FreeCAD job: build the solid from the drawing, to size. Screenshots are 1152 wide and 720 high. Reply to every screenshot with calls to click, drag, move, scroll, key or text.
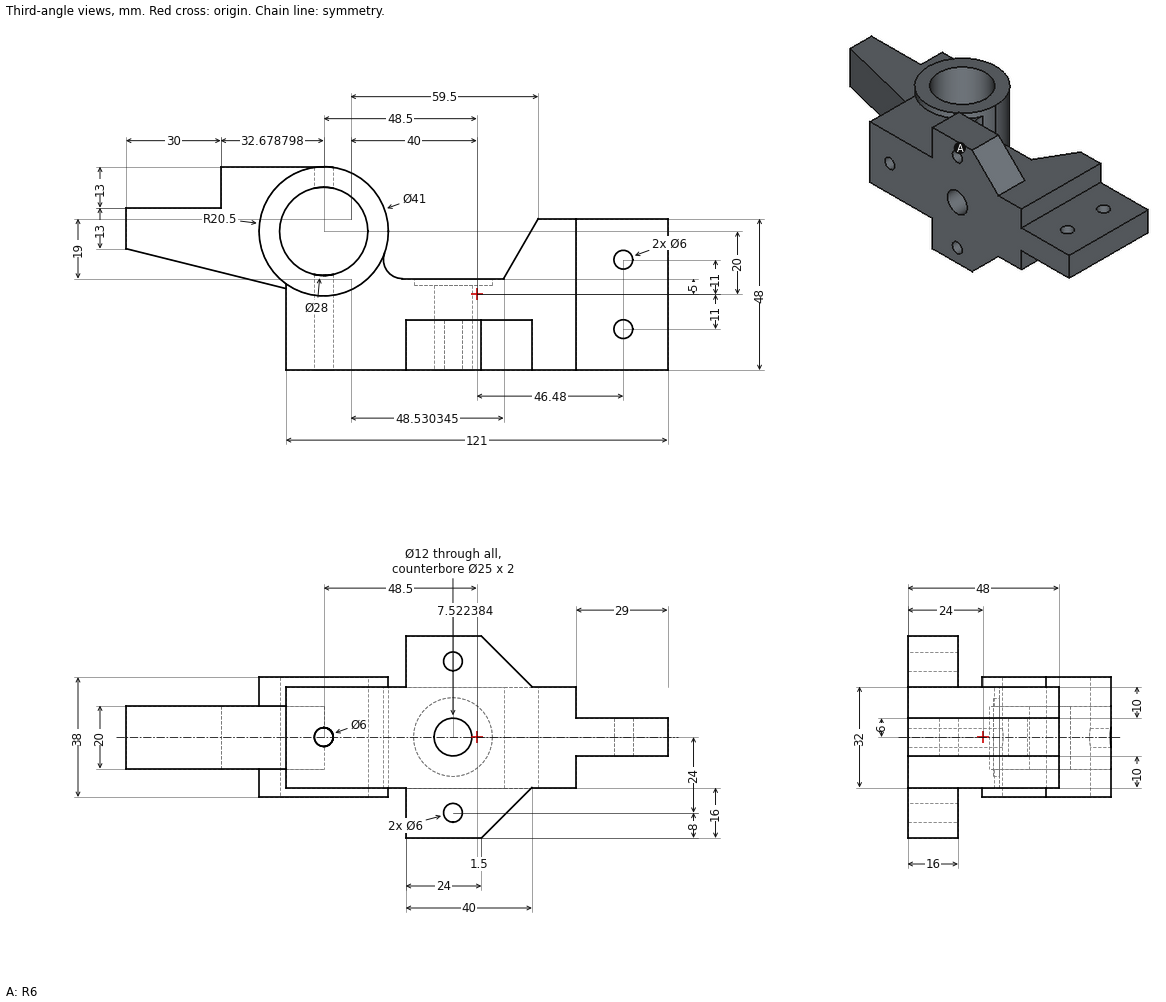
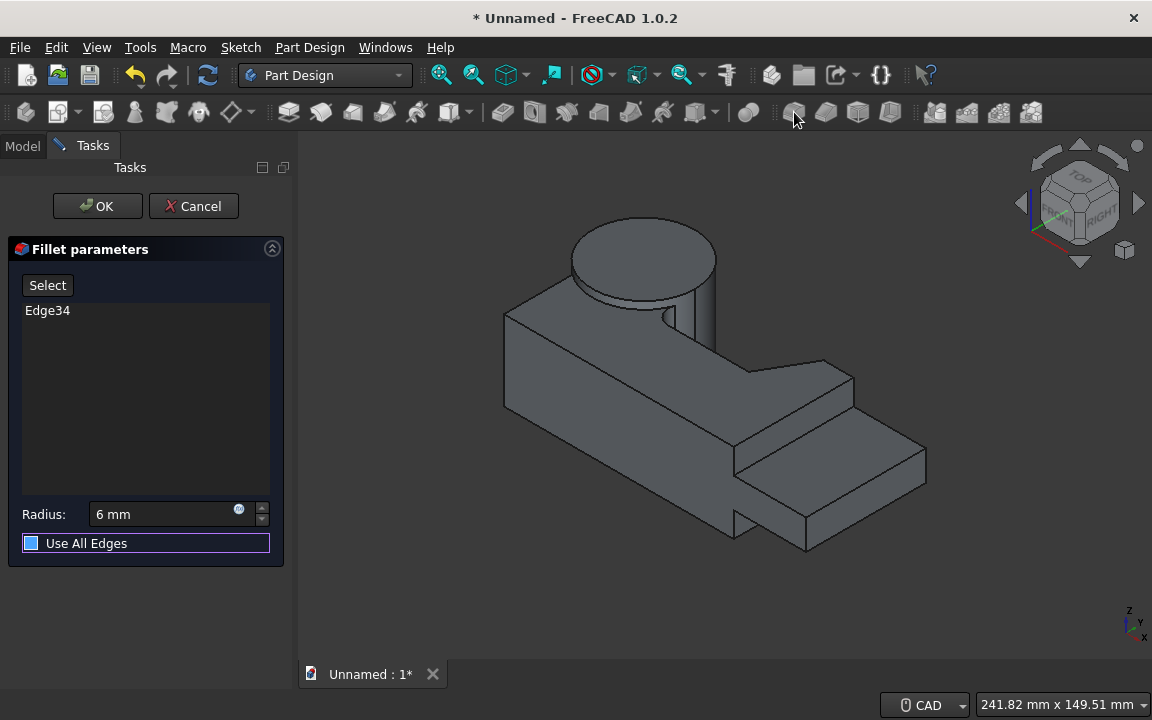
click(98, 206)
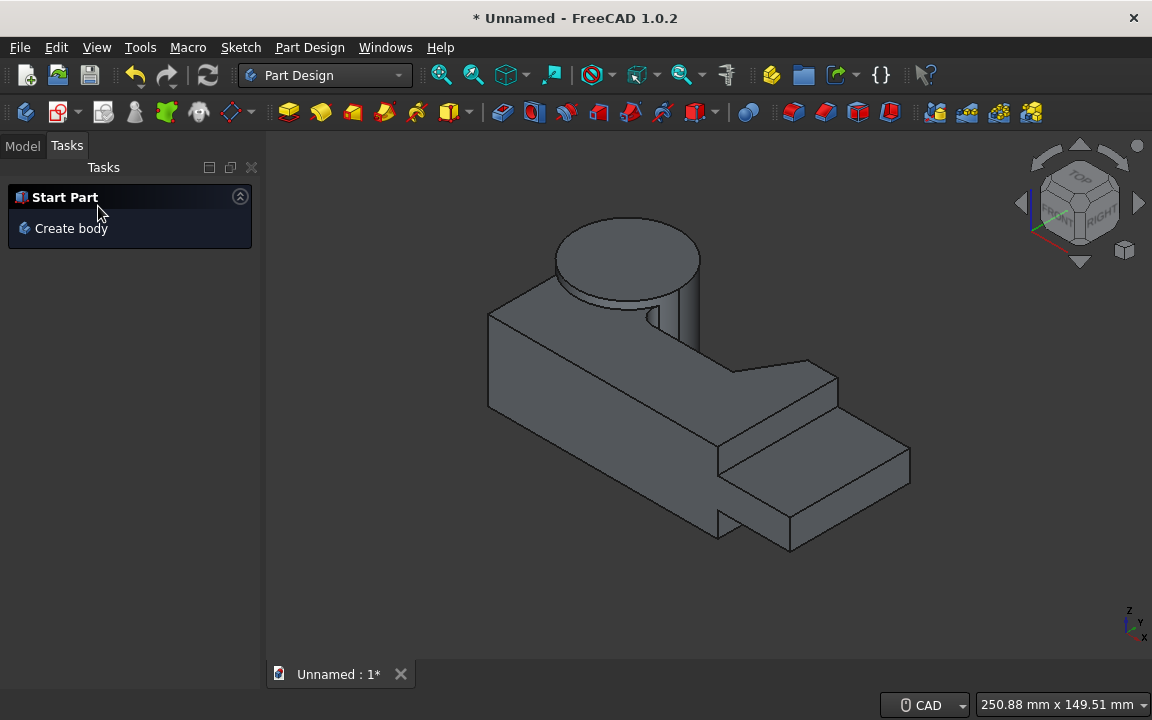
click(58, 112)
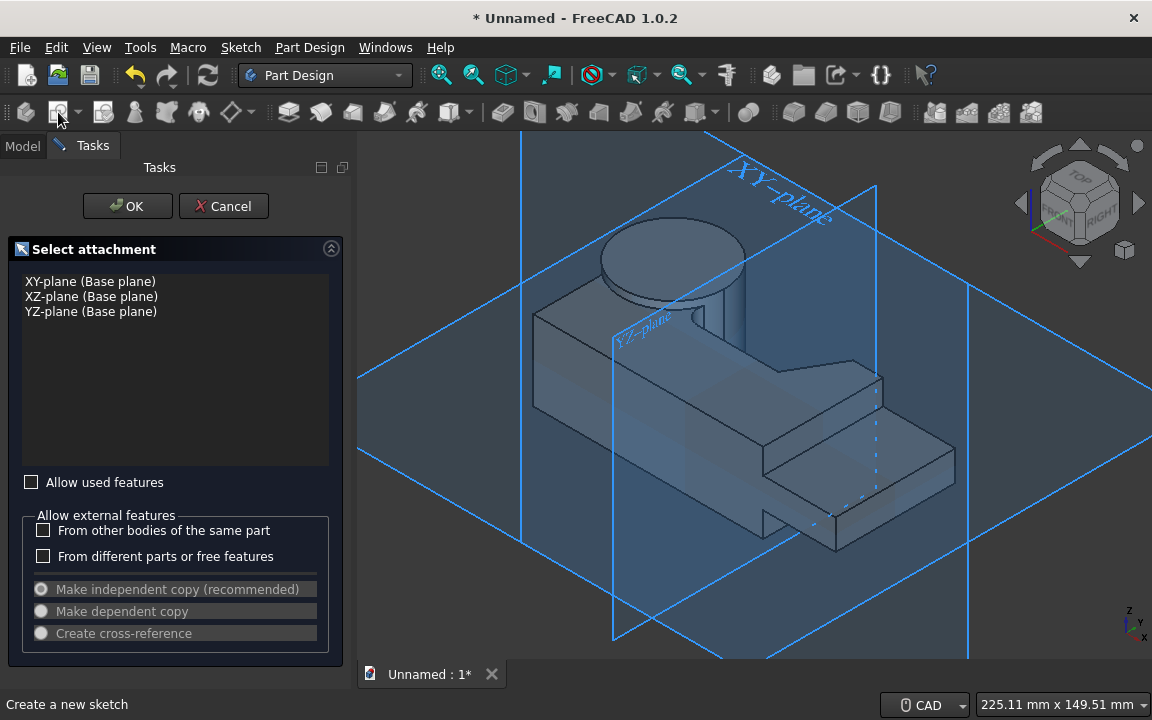
click(82, 282)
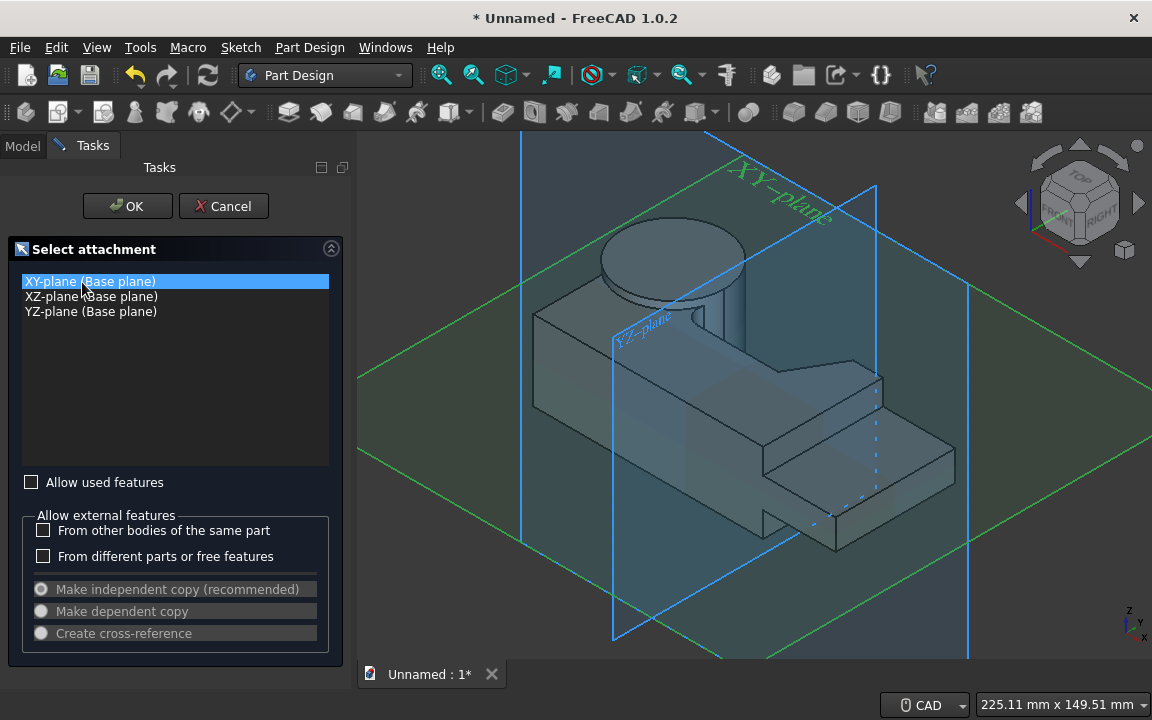
click(128, 206)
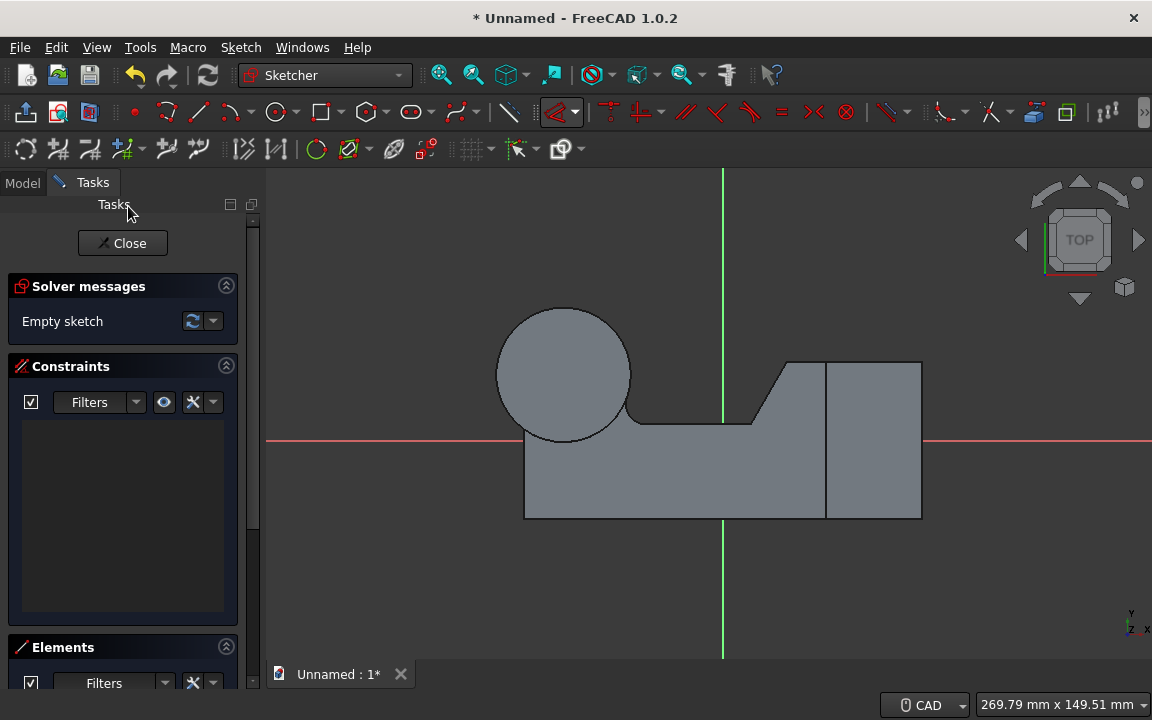
key(q)
key(s)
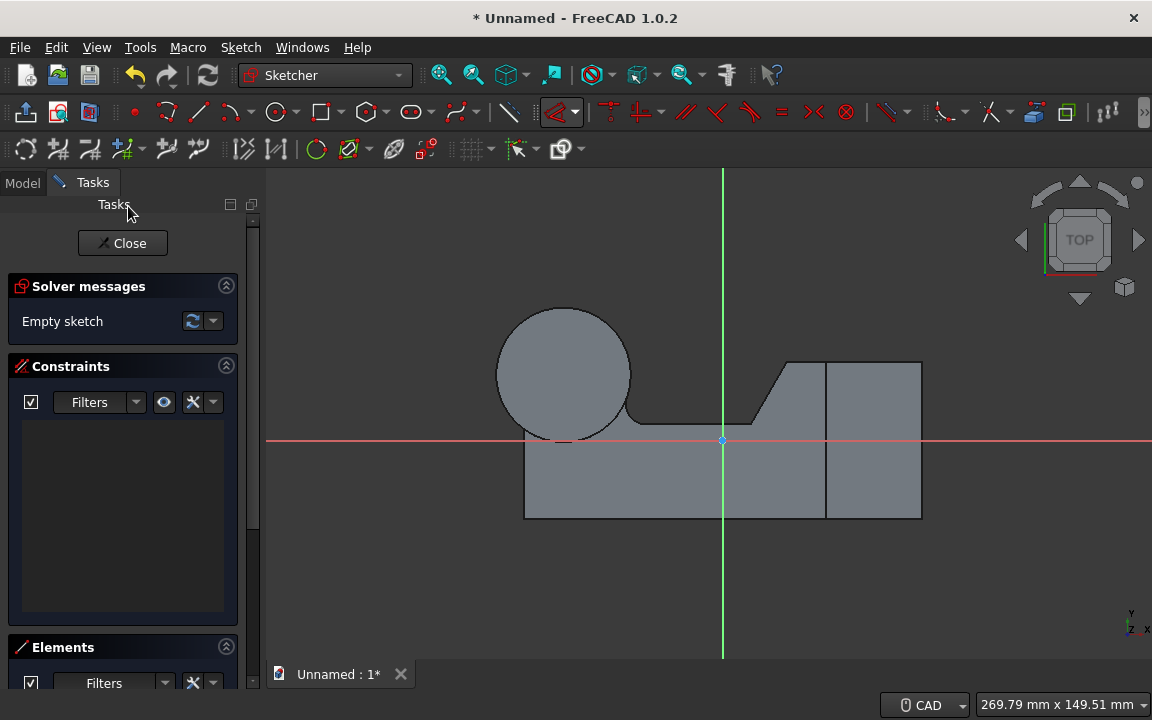
key(g)
key(m)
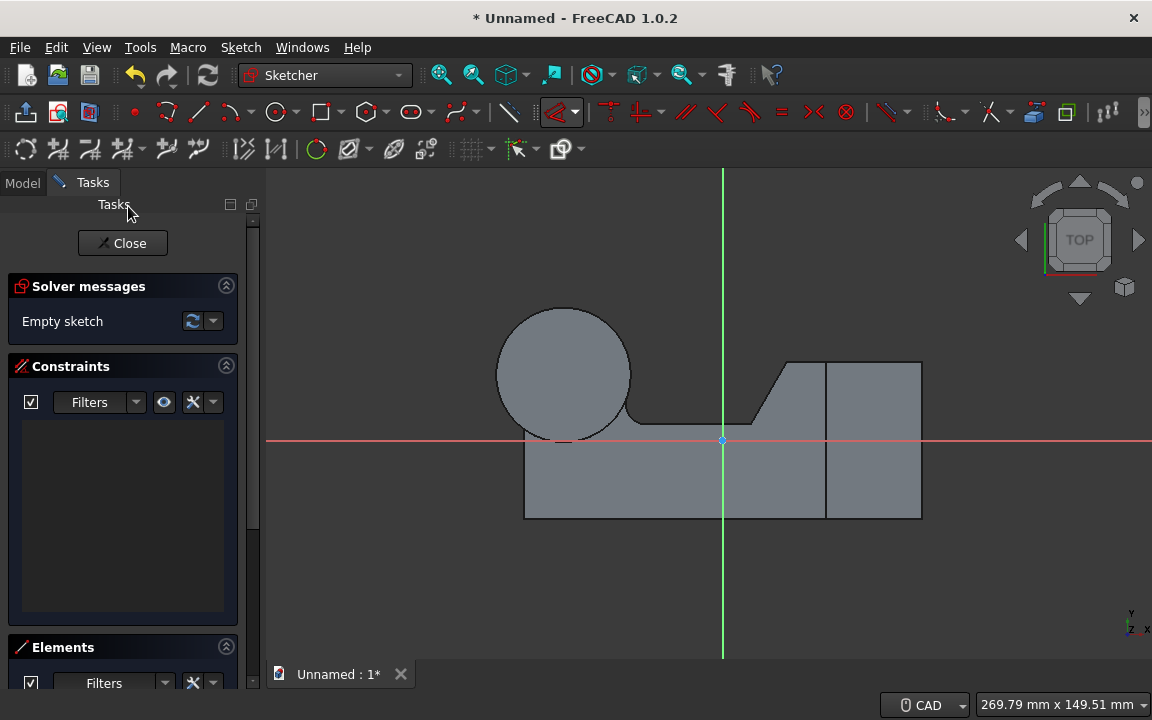
click(564, 308)
click(456, 308)
click(456, 350)
click(358, 350)
click(358, 393)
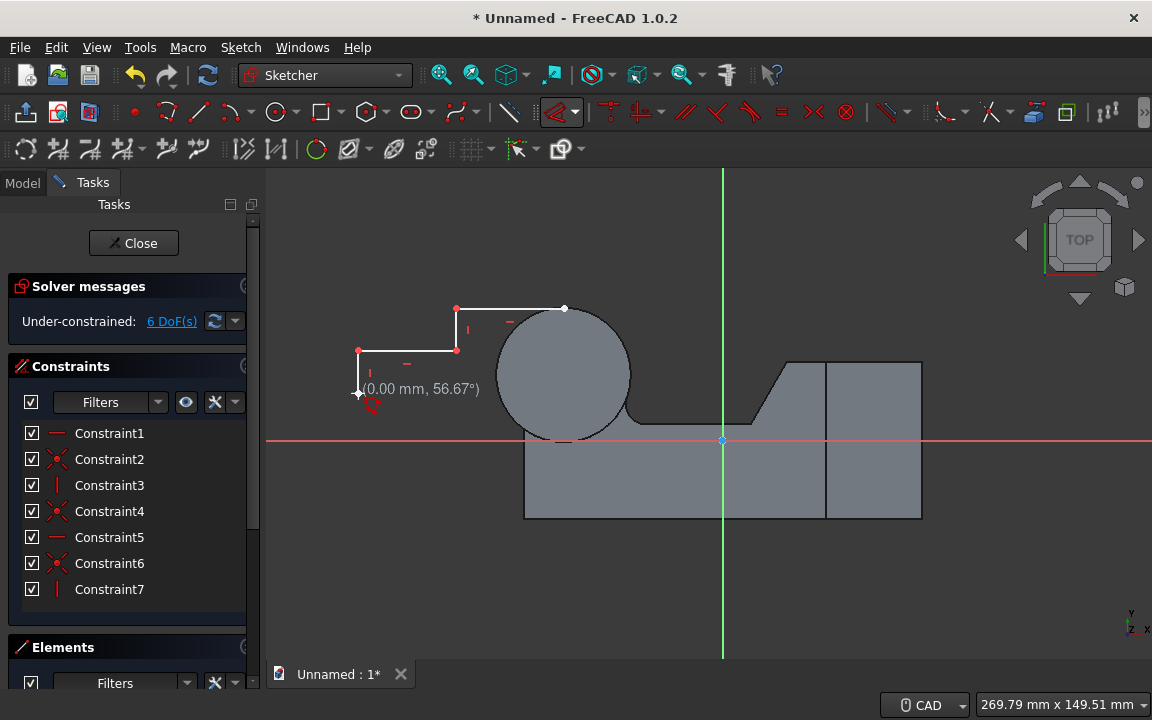
scroll(547, 440, up, 19)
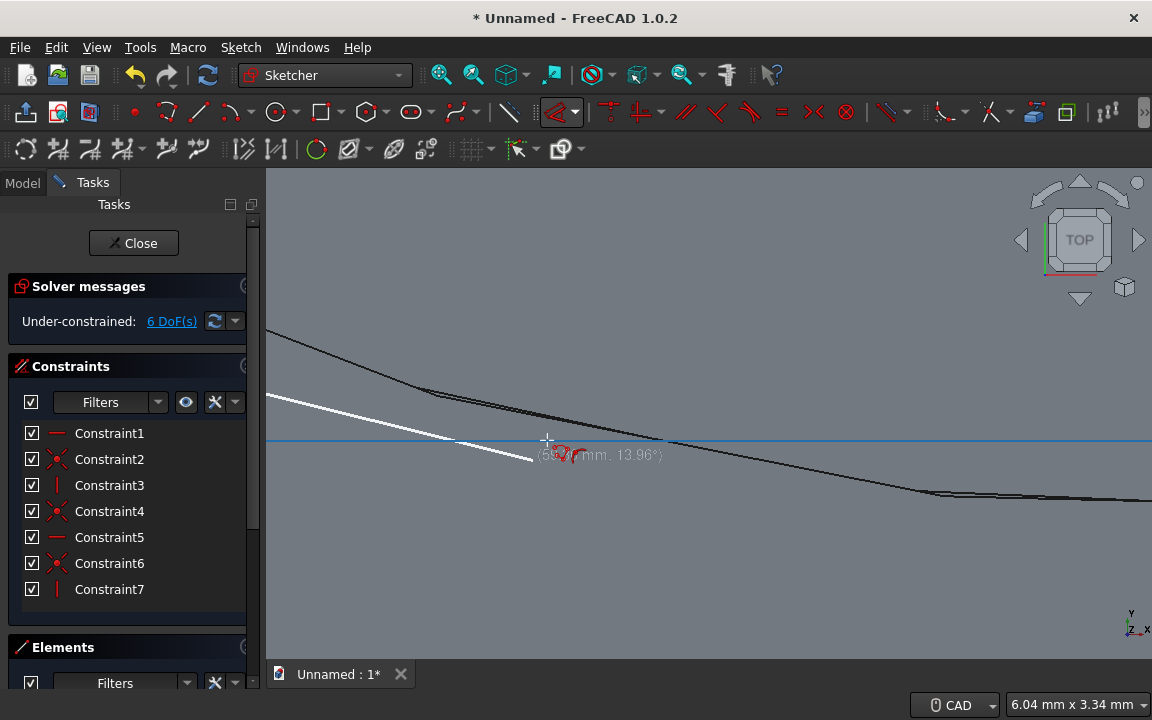
click(545, 425)
right_click(545, 425)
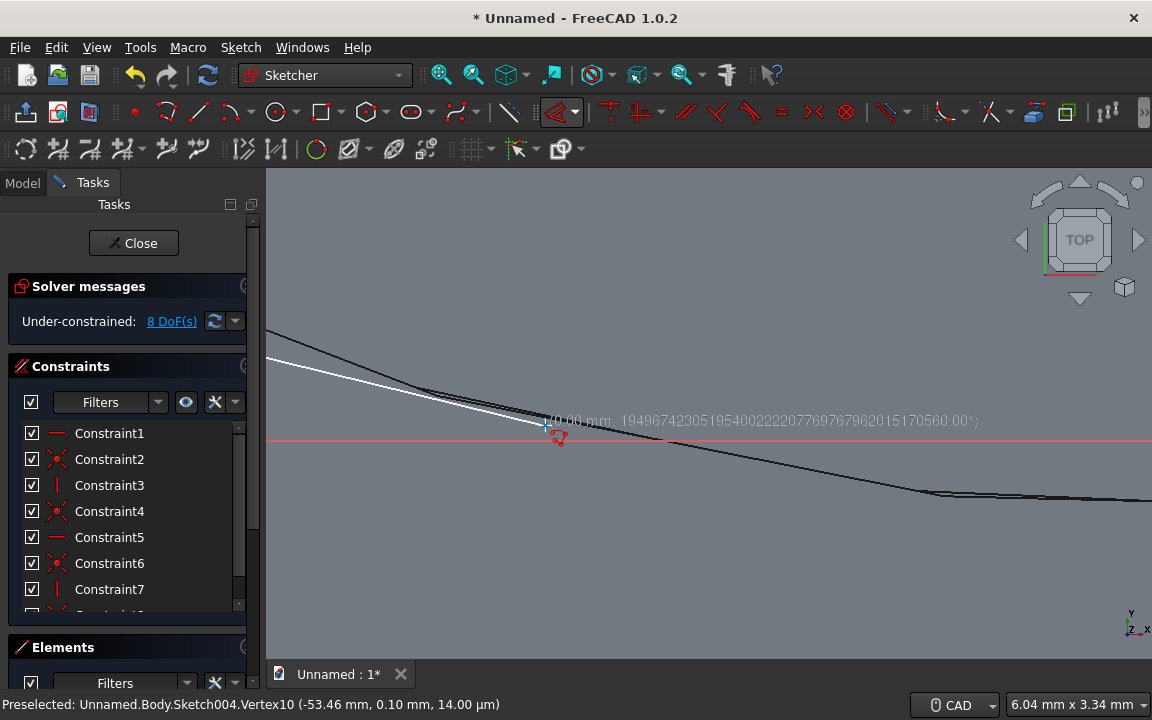
key(g)
key(3)
key(a)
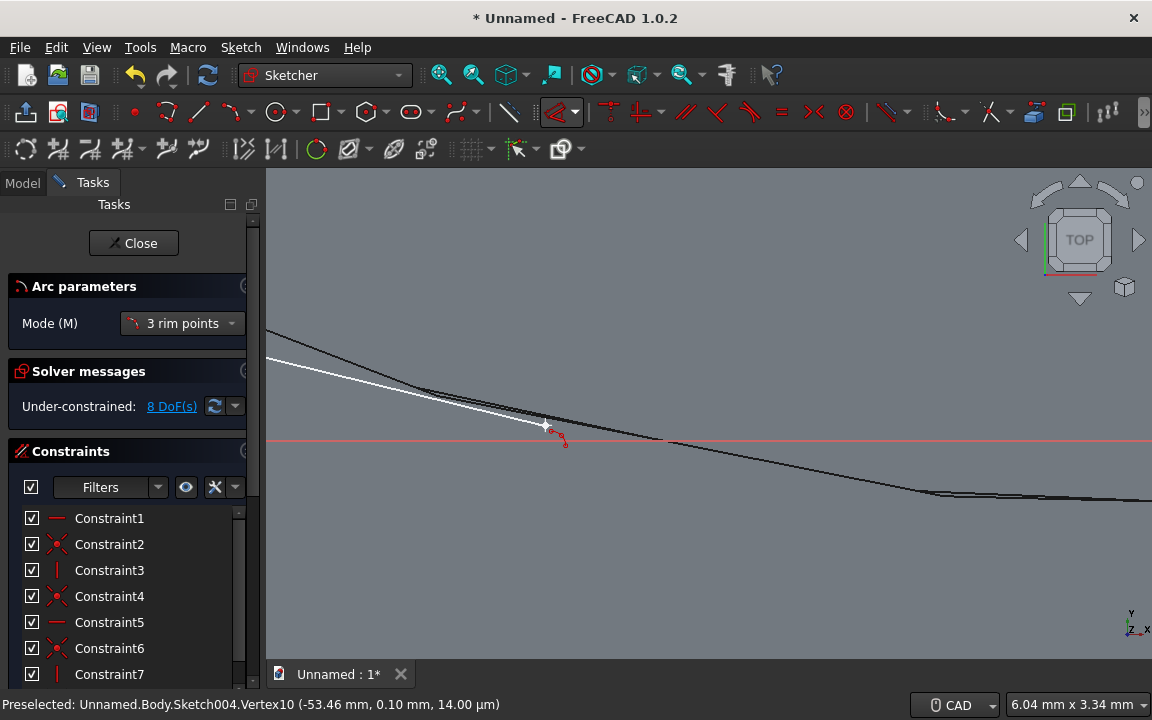
click(545, 426)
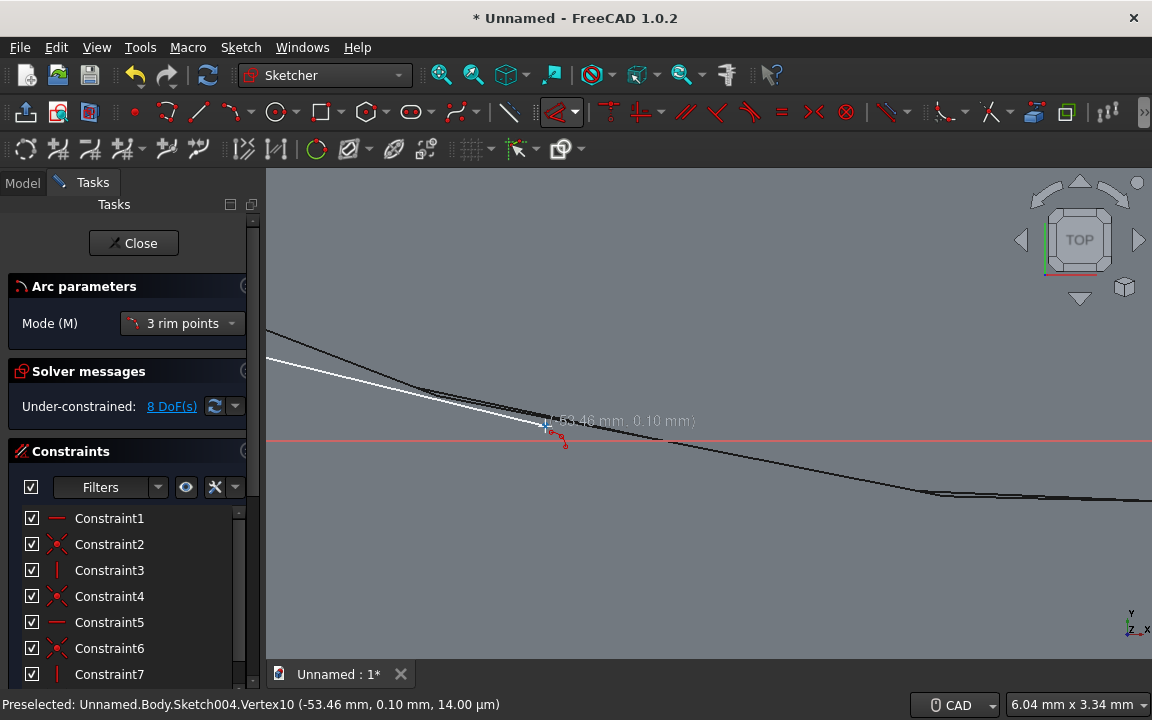
scroll(655, 515, down, 17)